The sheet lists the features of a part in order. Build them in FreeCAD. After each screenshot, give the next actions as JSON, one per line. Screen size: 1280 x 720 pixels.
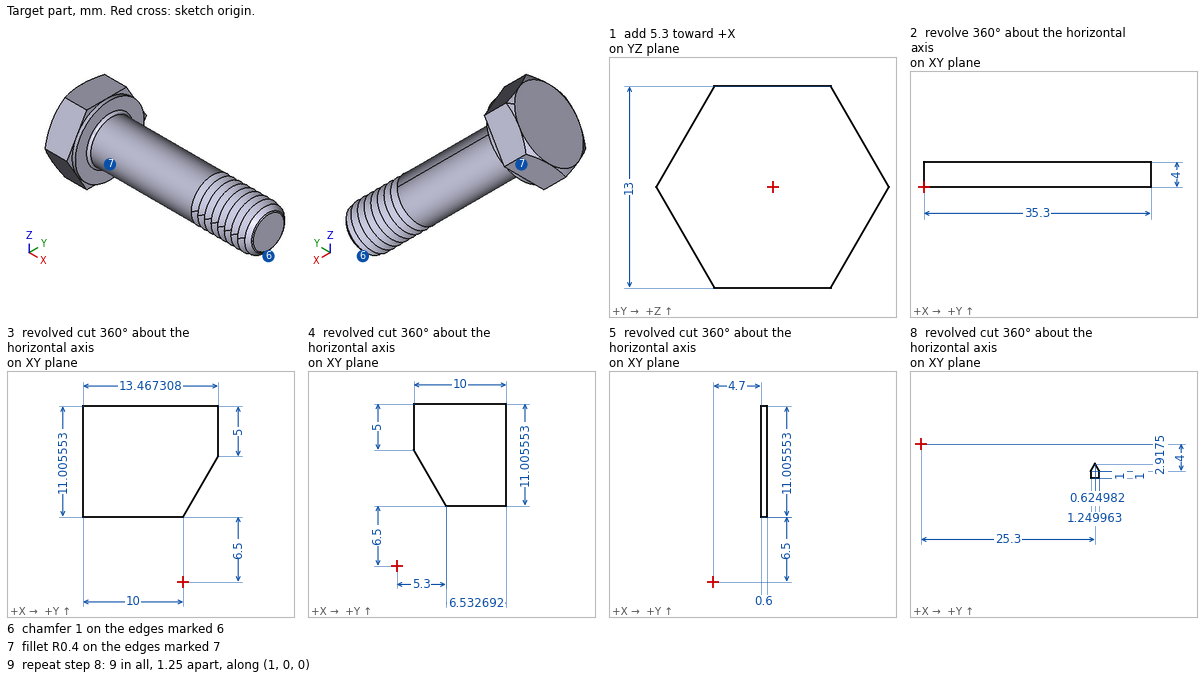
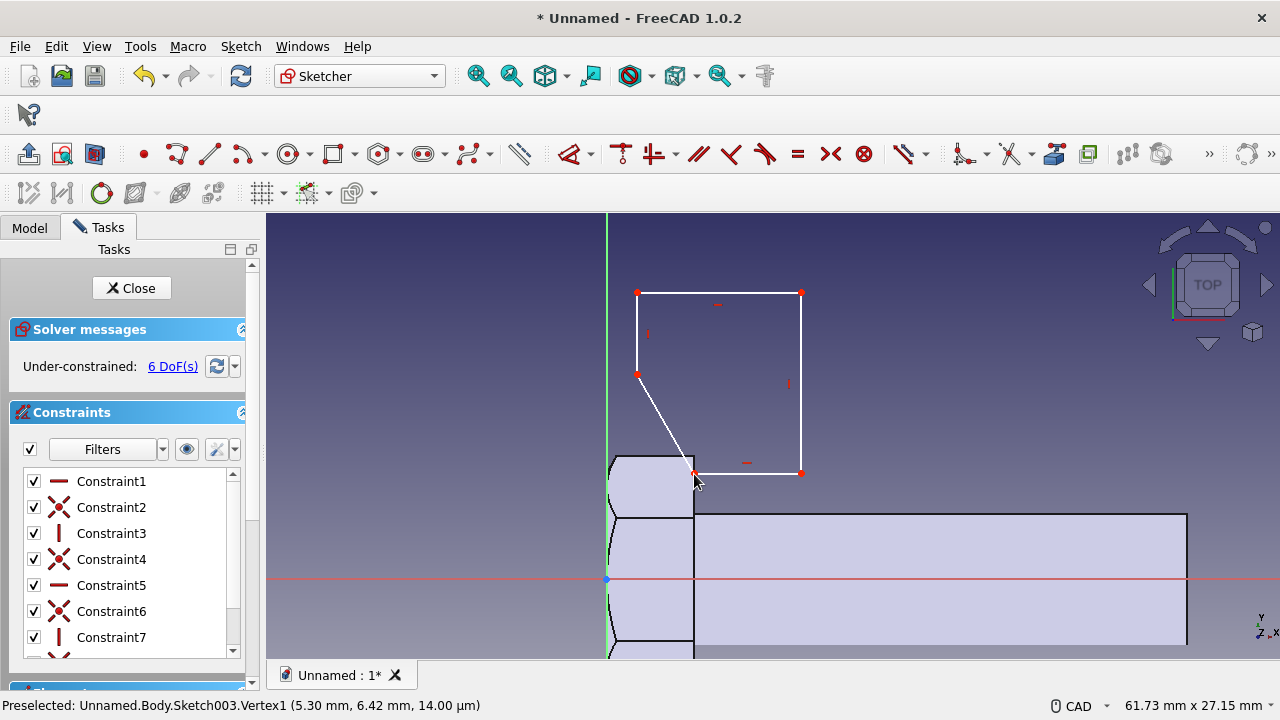
{"action": "left_click", "coordinate": [568, 154]}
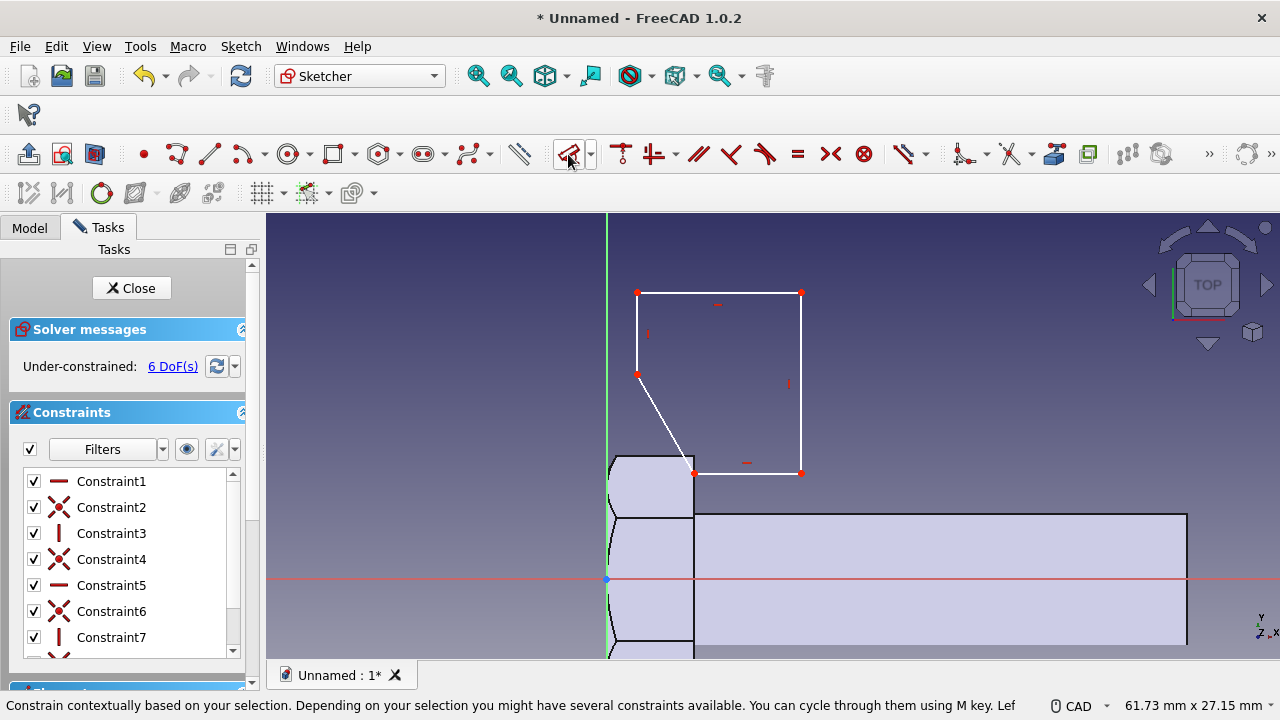
{"action": "left_click", "coordinate": [637, 318]}
{"action": "left_click", "coordinate": [671, 334]}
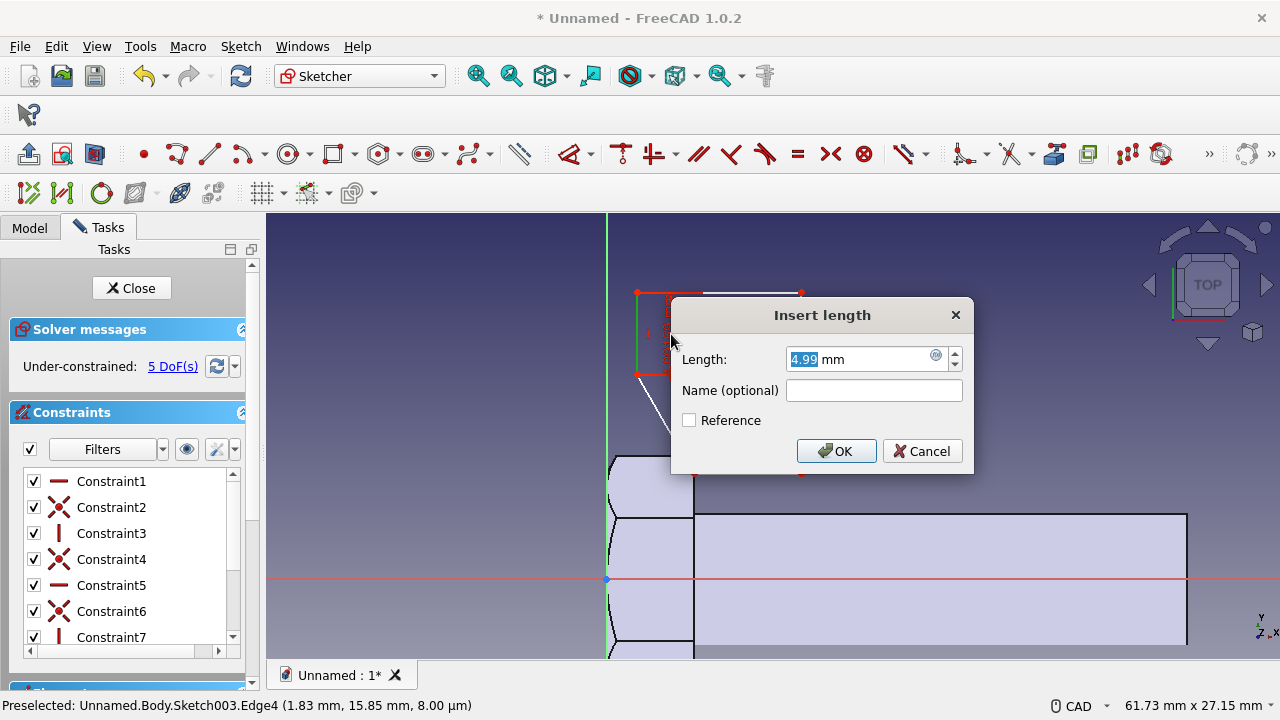
{"action": "type", "text": "5"}
{"action": "key", "text": "Return"}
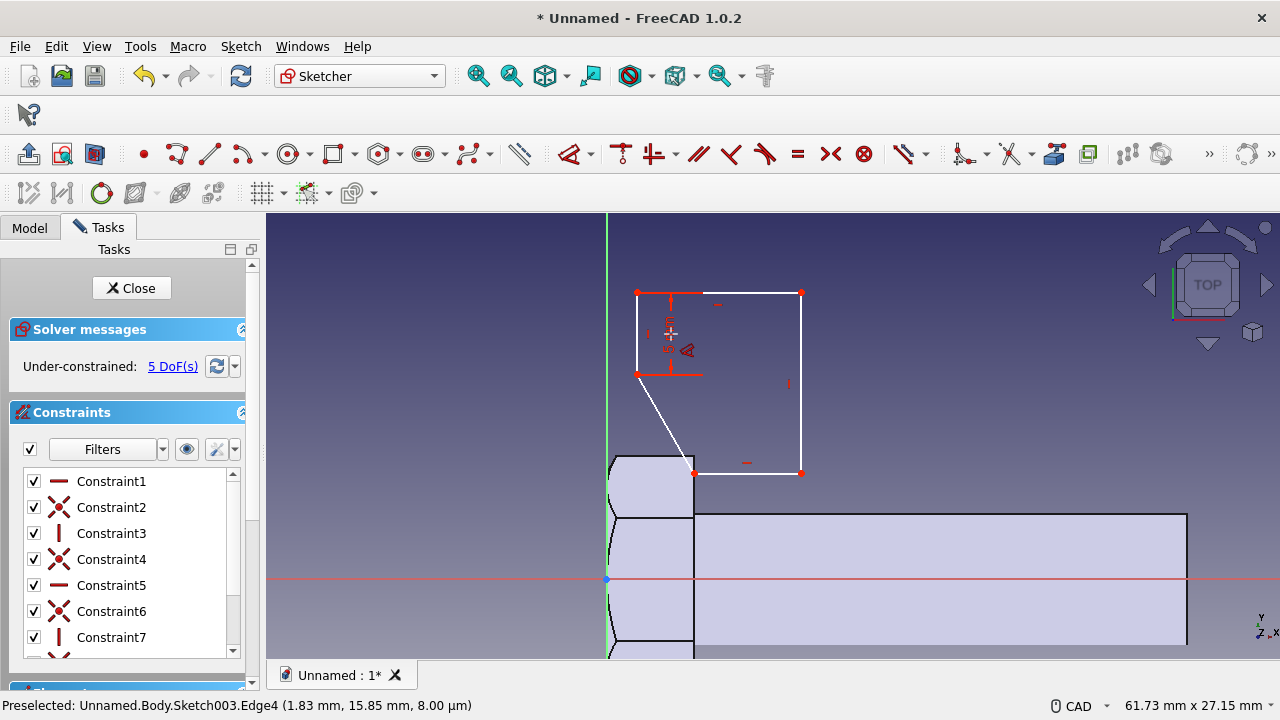
{"action": "left_click", "coordinate": [752, 293]}
{"action": "left_click", "coordinate": [719, 259]}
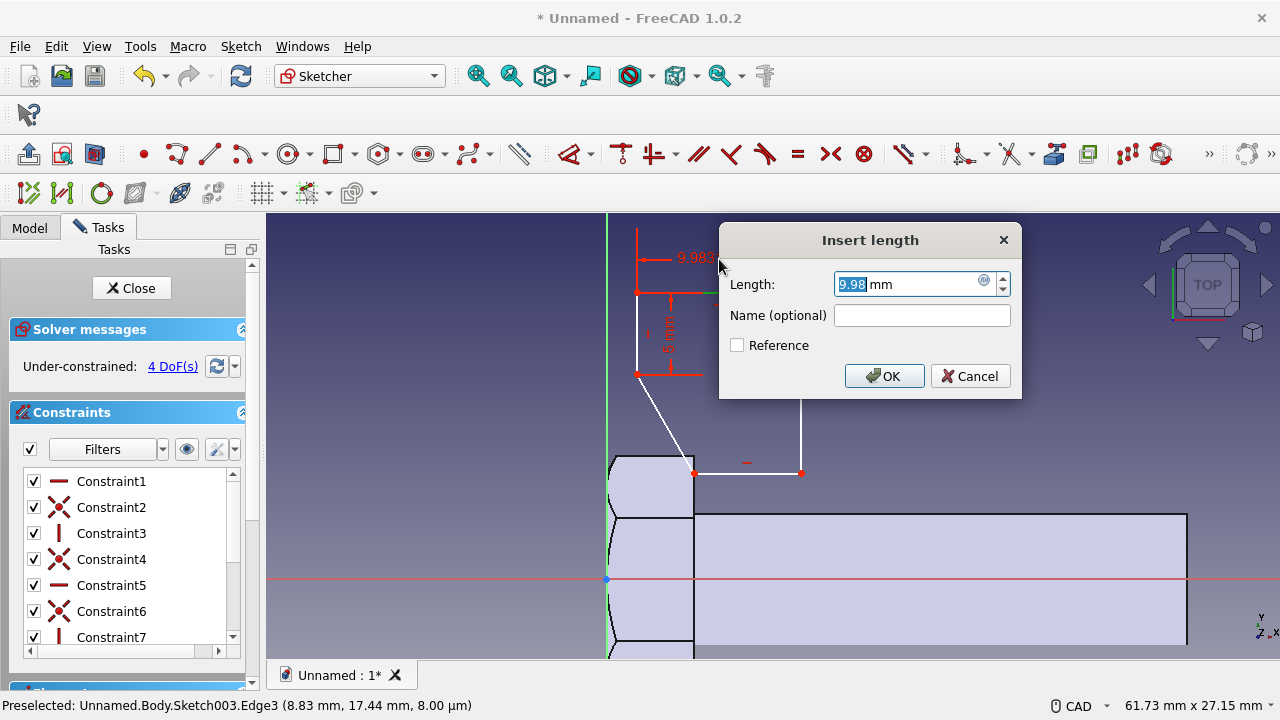
{"action": "type", "text": "10"}
{"action": "key", "text": "Return"}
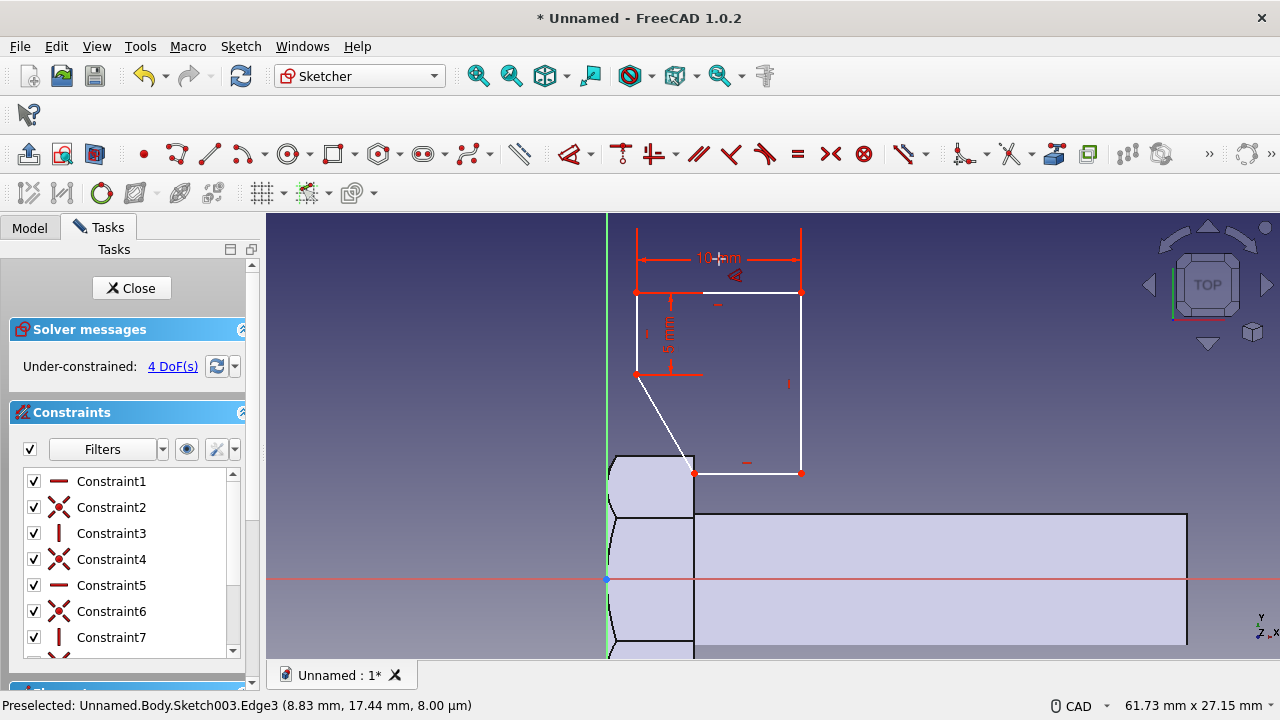
{"action": "left_click", "coordinate": [694, 474]}
{"action": "left_click", "coordinate": [650, 613]}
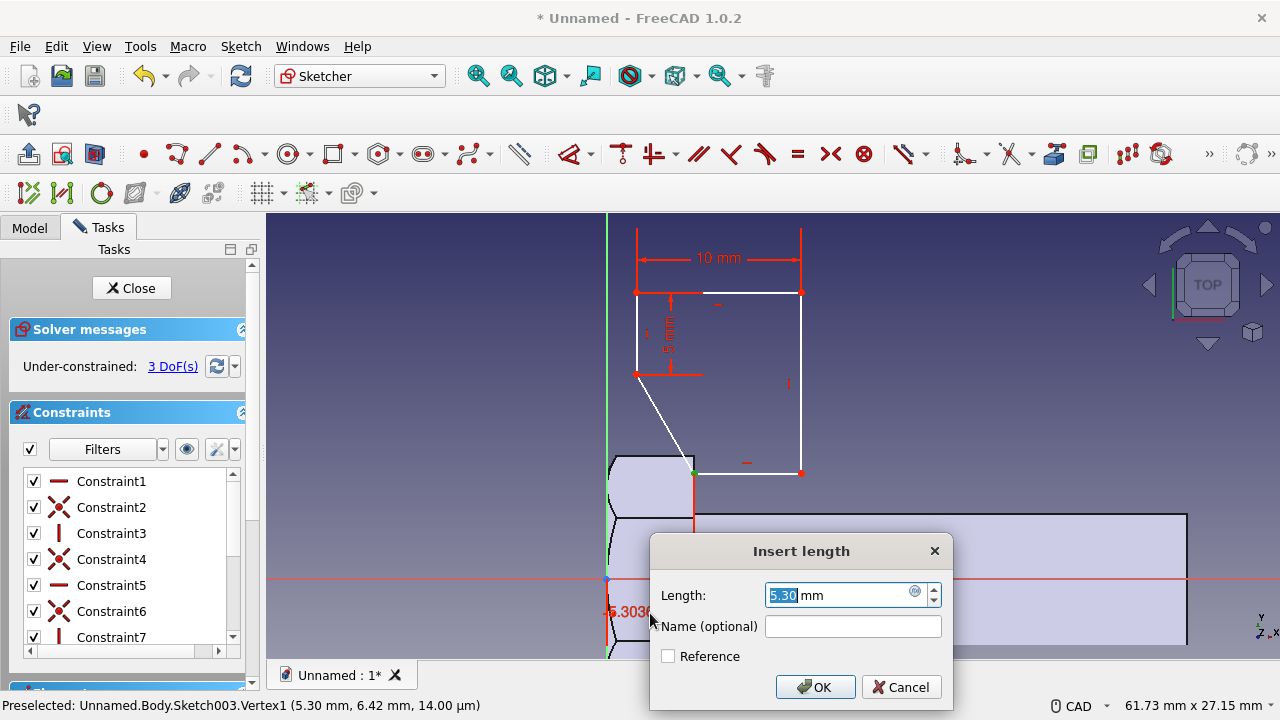
{"action": "type", "text": "5.3"}
{"action": "key", "text": "Return"}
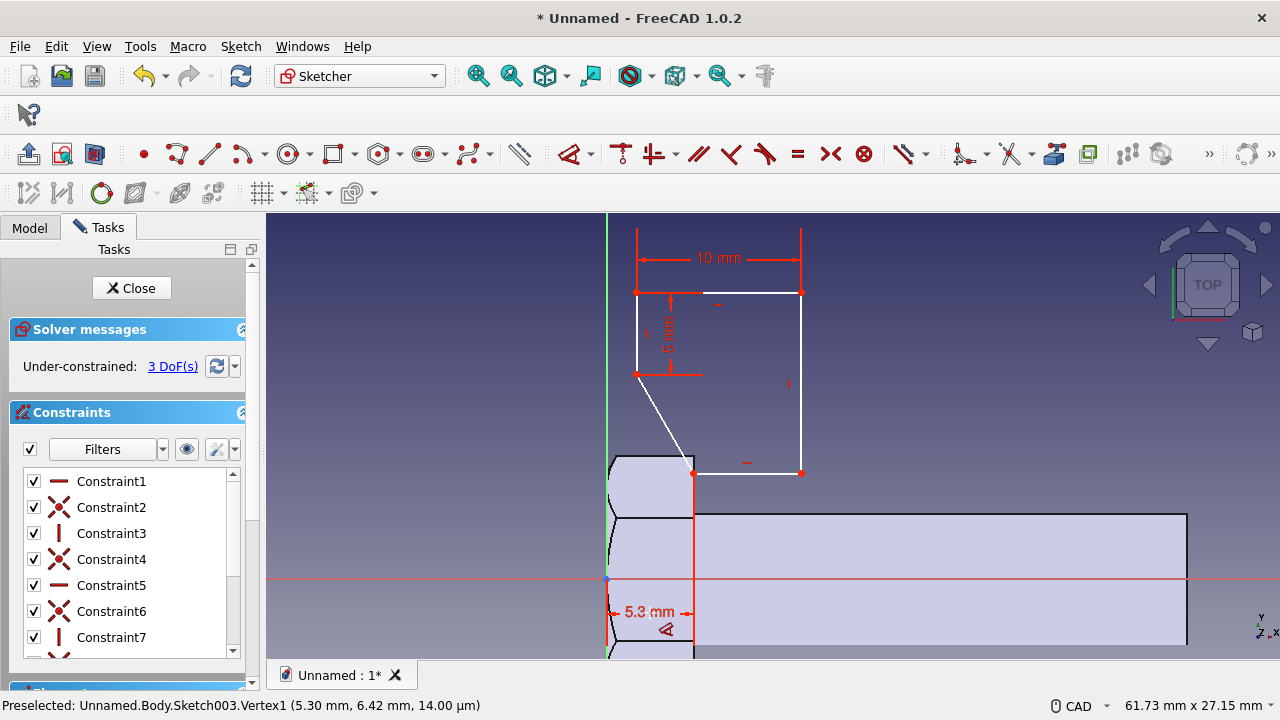
{"action": "left_click", "coordinate": [694, 474]}
{"action": "left_click", "coordinate": [573, 527]}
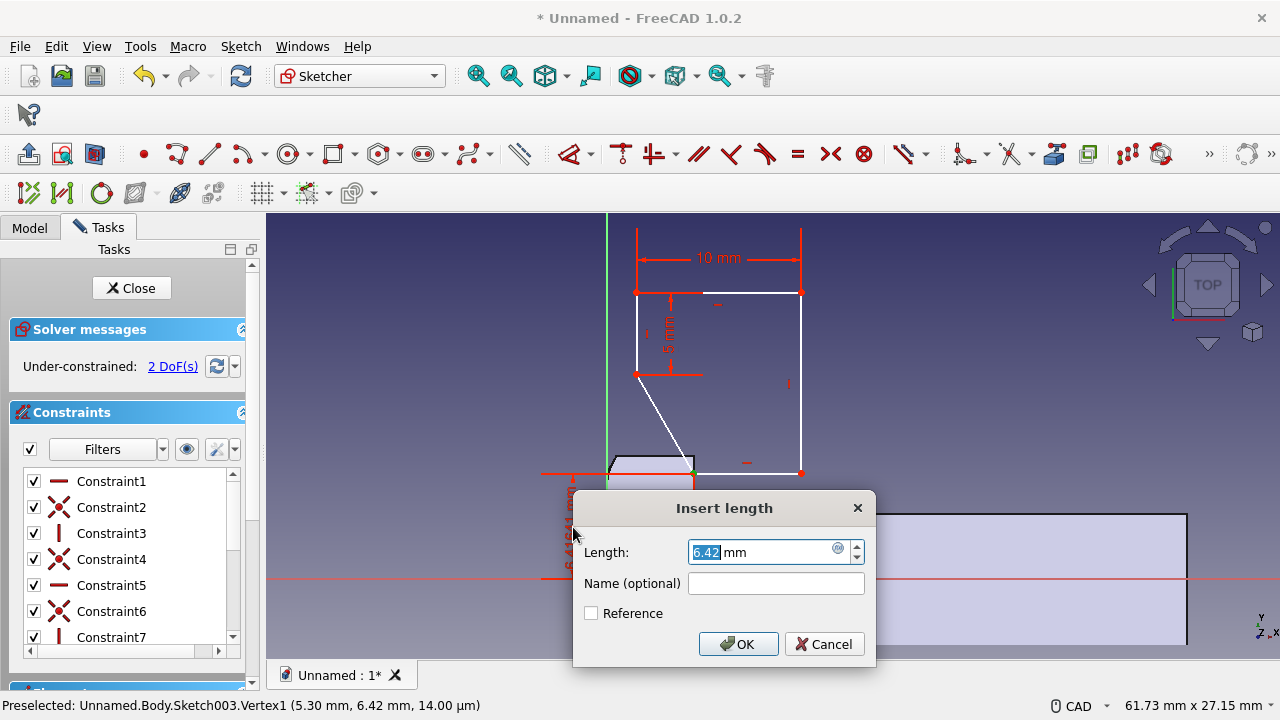
{"action": "type", "text": "6.5"}
{"action": "key", "text": "Return"}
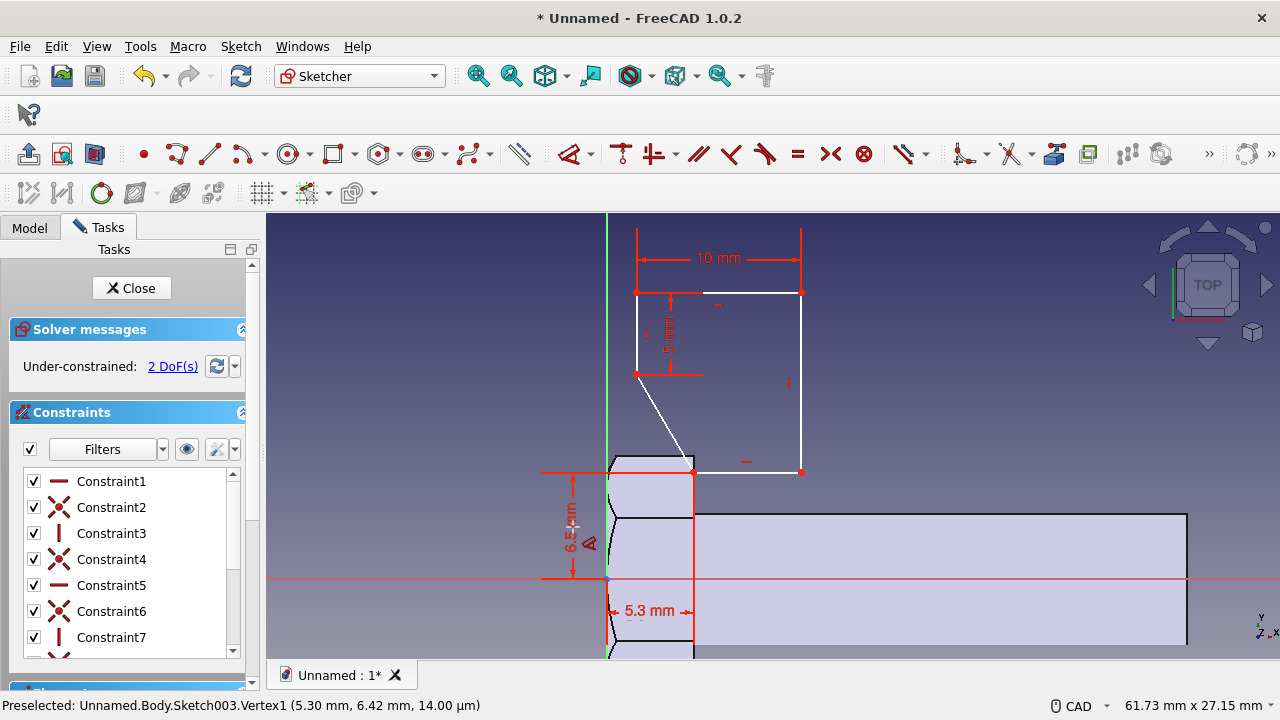
{"action": "left_click", "coordinate": [726, 473]}
{"action": "left_click", "coordinate": [747, 507]}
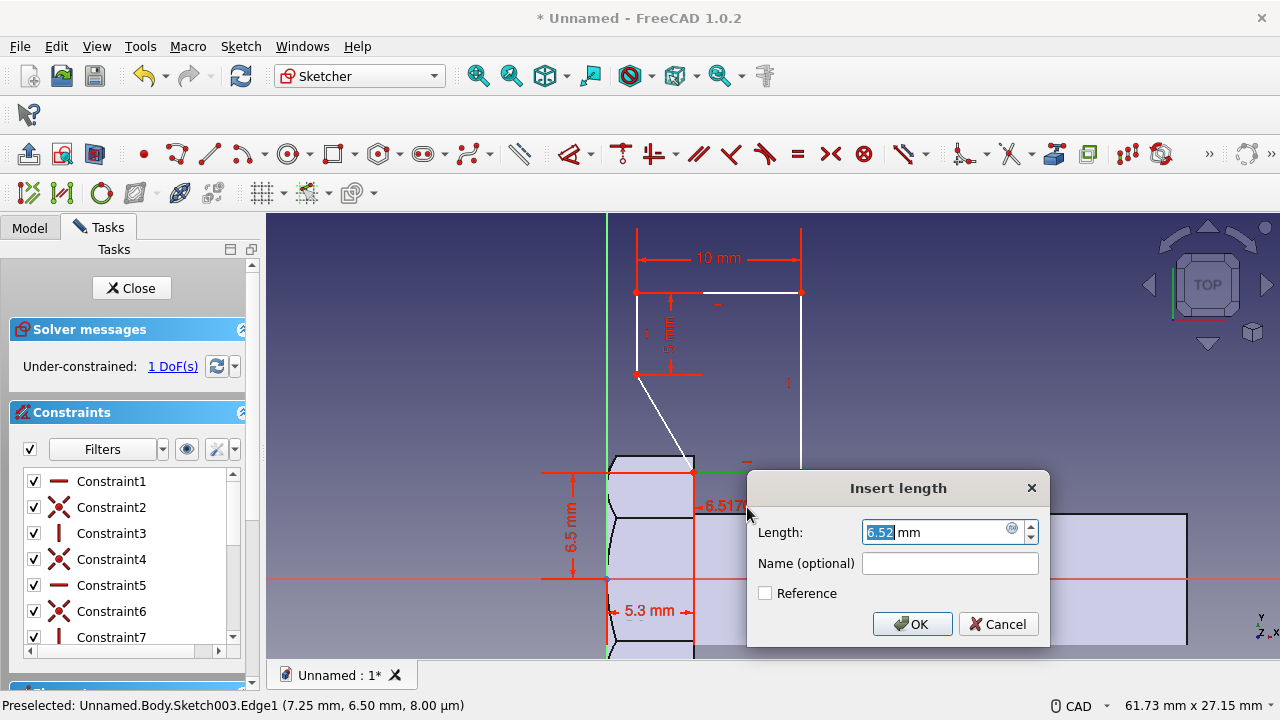
{"action": "type", "text": "6.532692"}
{"action": "key", "text": "Return"}